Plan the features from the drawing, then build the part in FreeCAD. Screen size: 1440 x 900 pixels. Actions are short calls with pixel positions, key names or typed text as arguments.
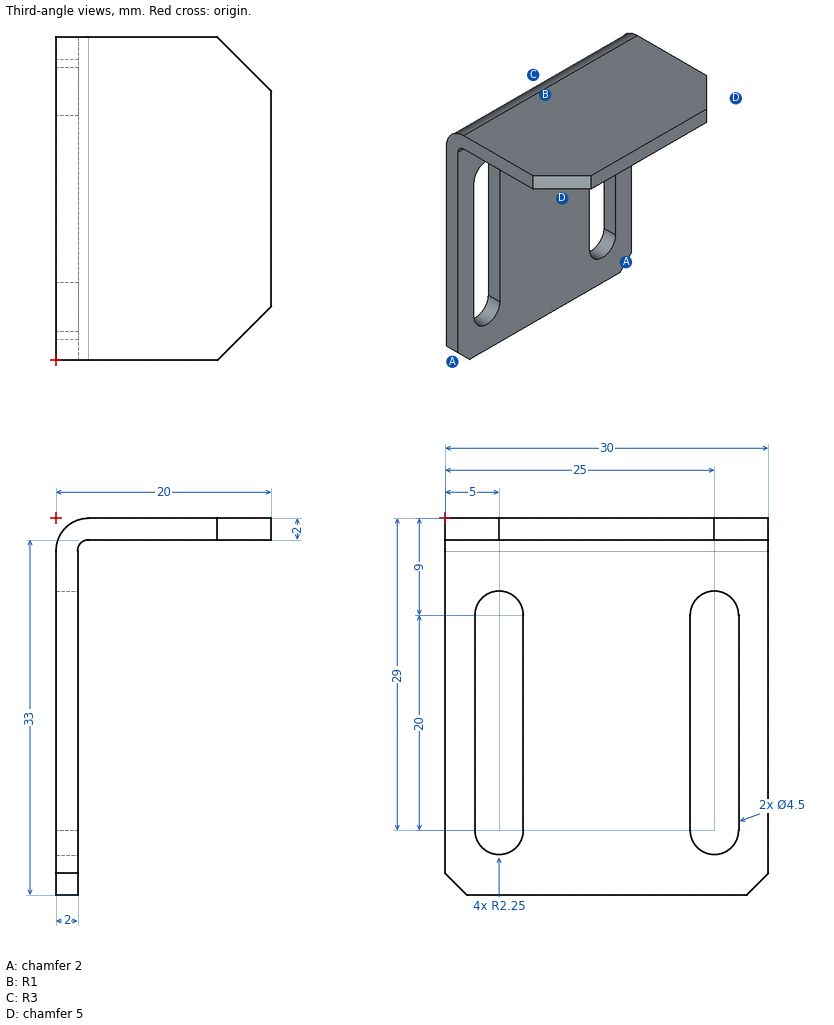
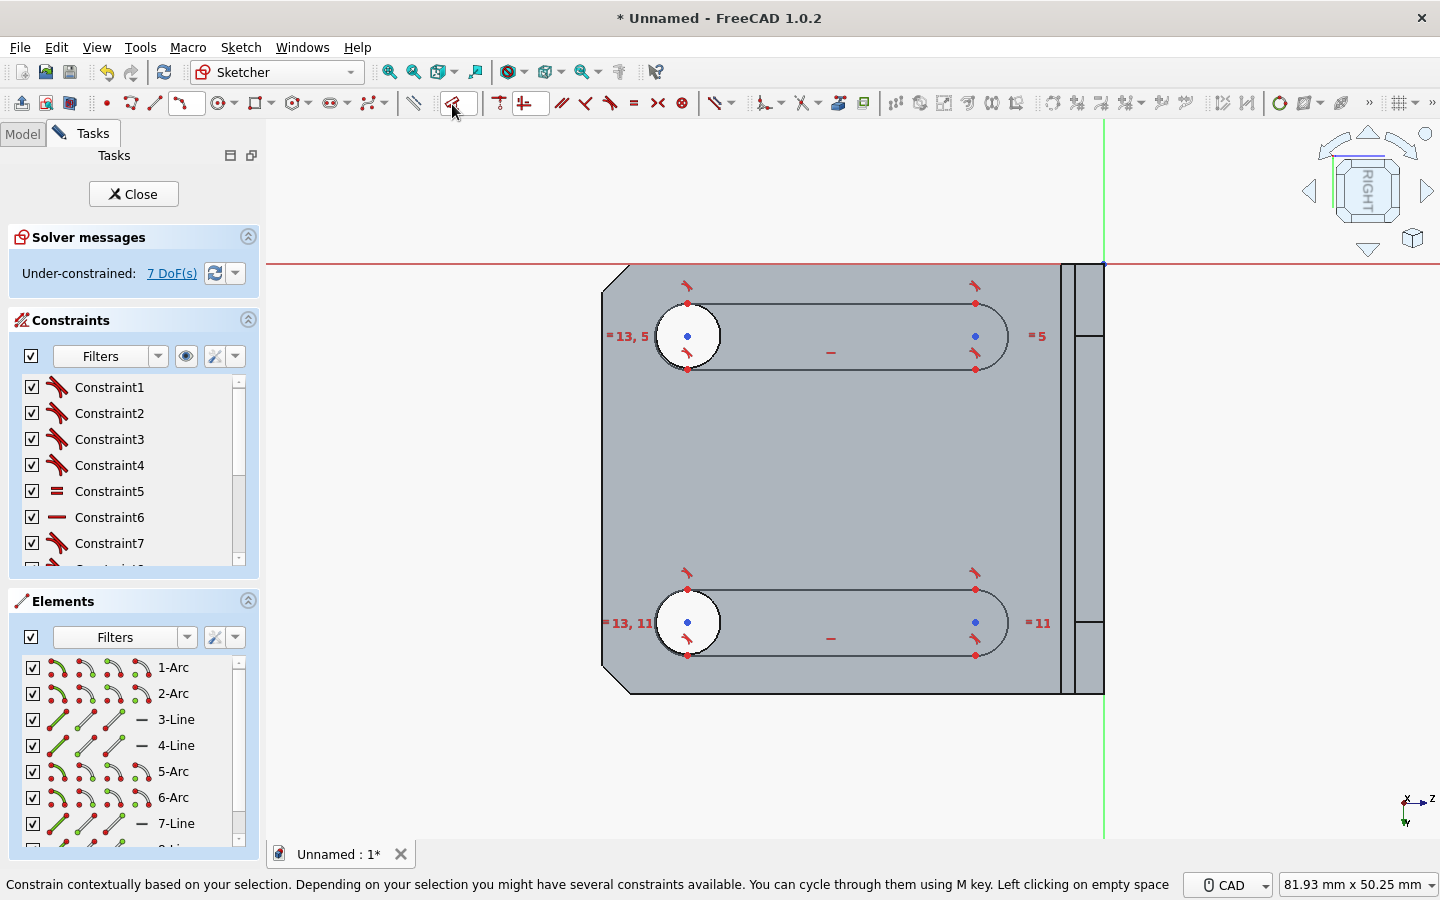
scroll(661, 318, up, 2)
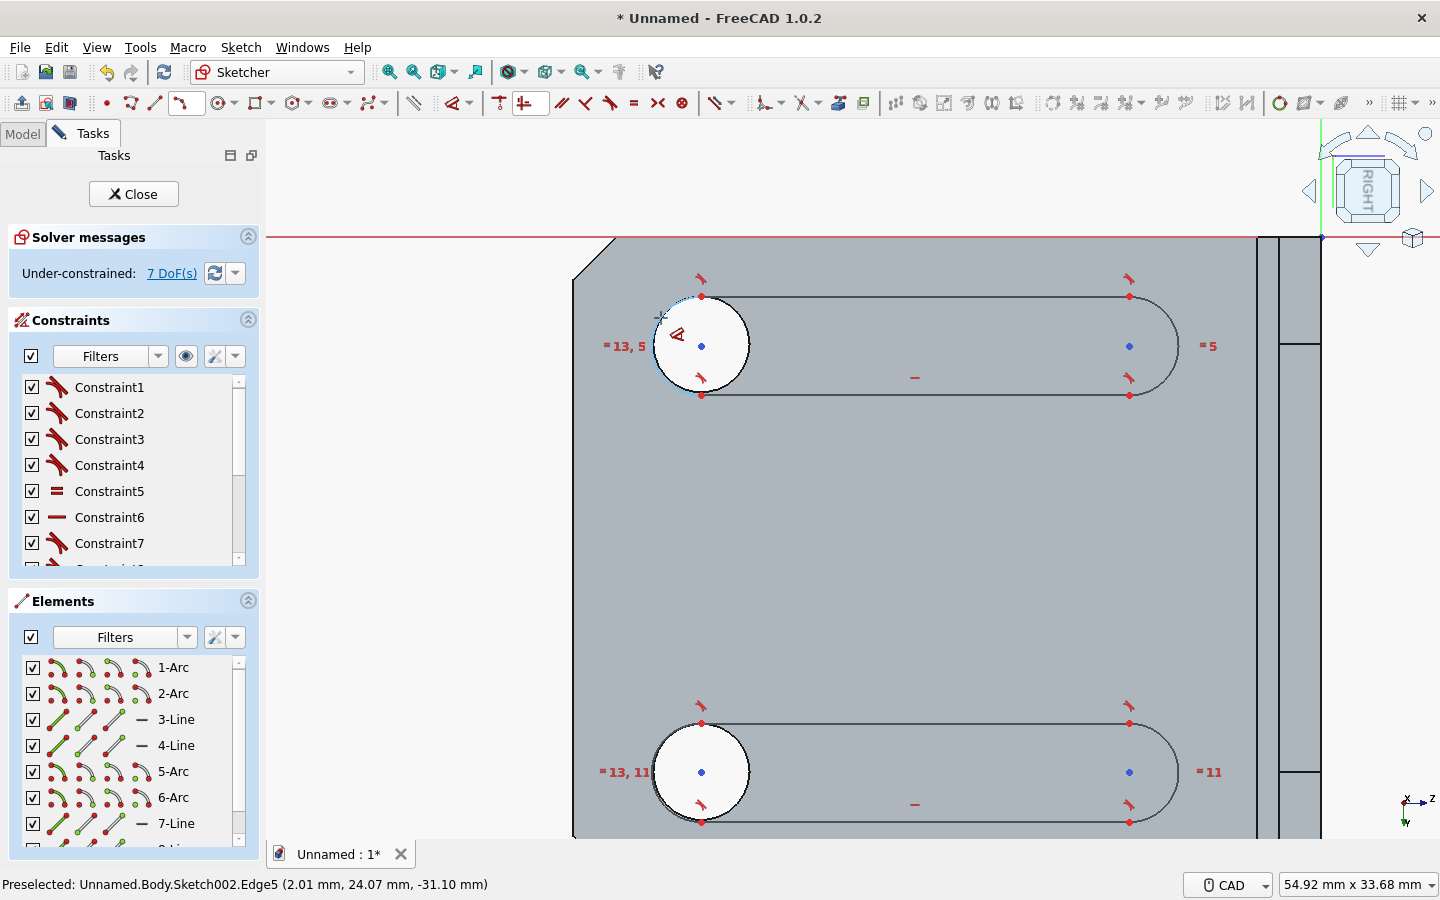
click(661, 317)
click(635, 298)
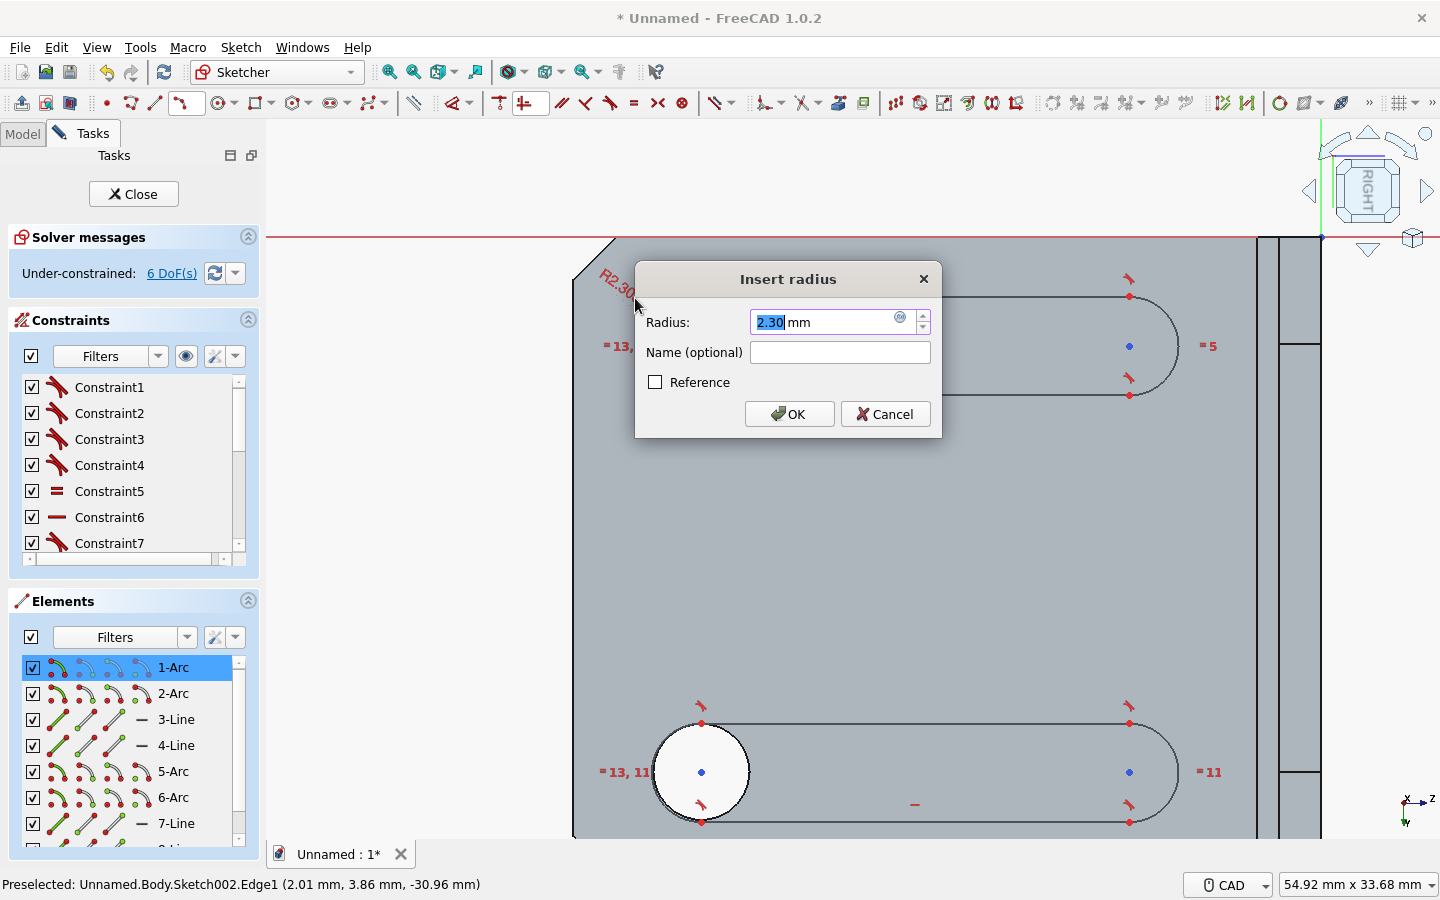
text(2.25)
key(Return)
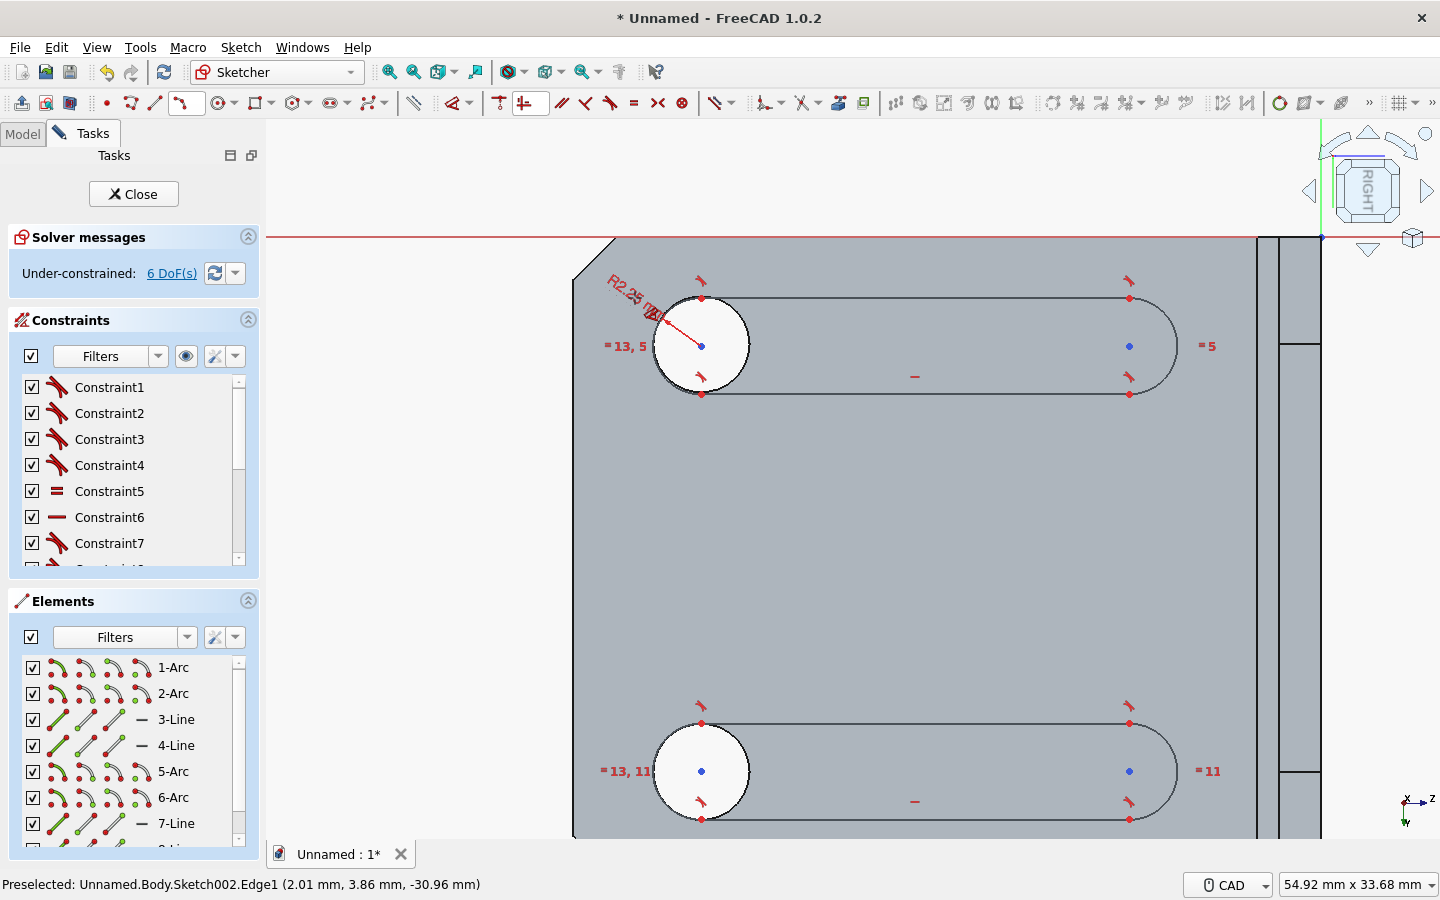
click(830, 298)
click(915, 264)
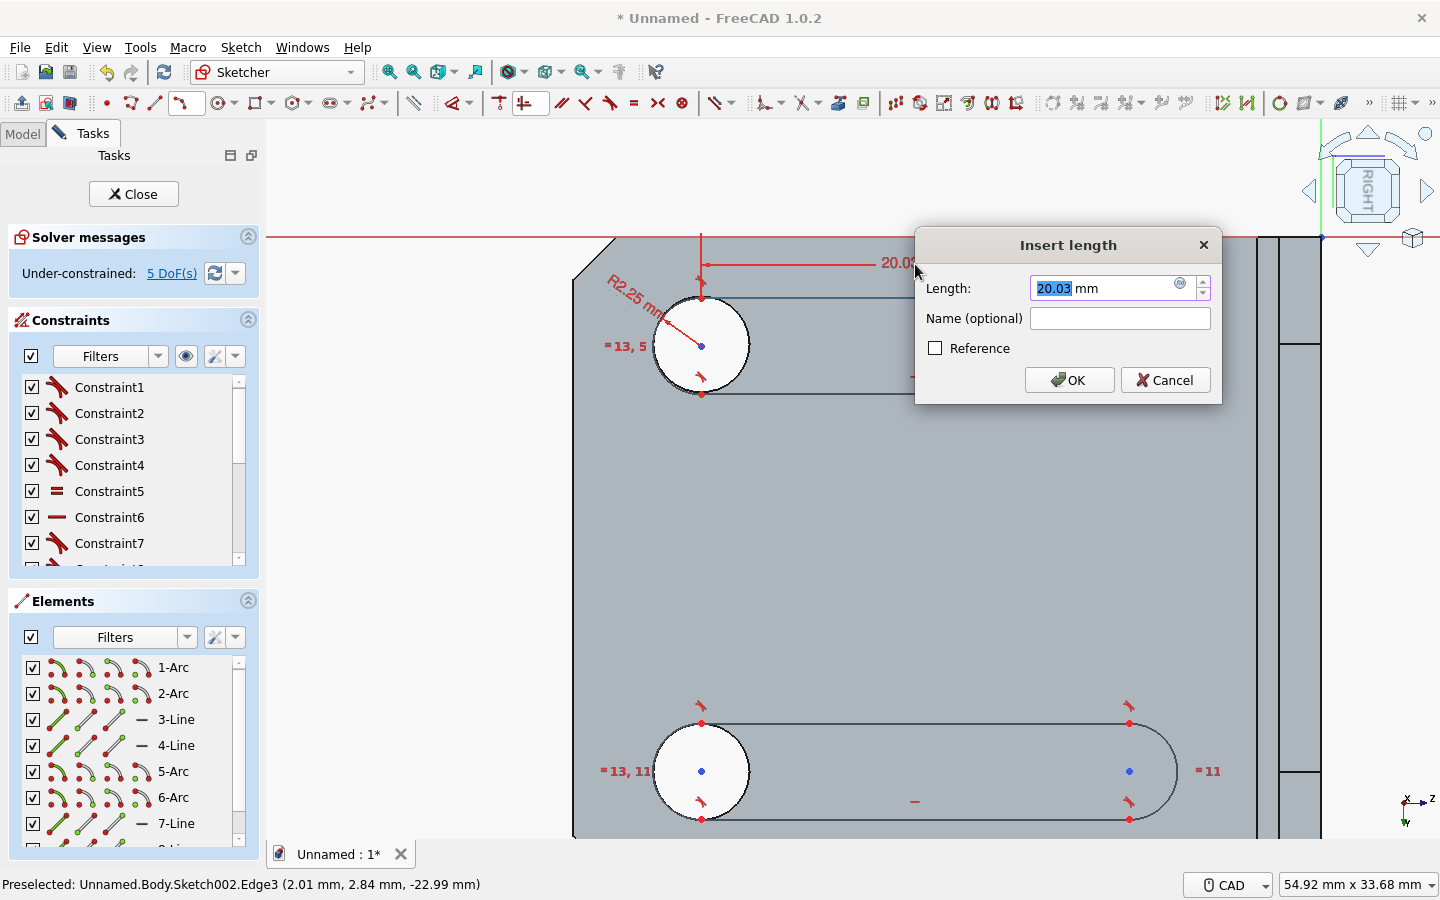
text(20)
key(Return)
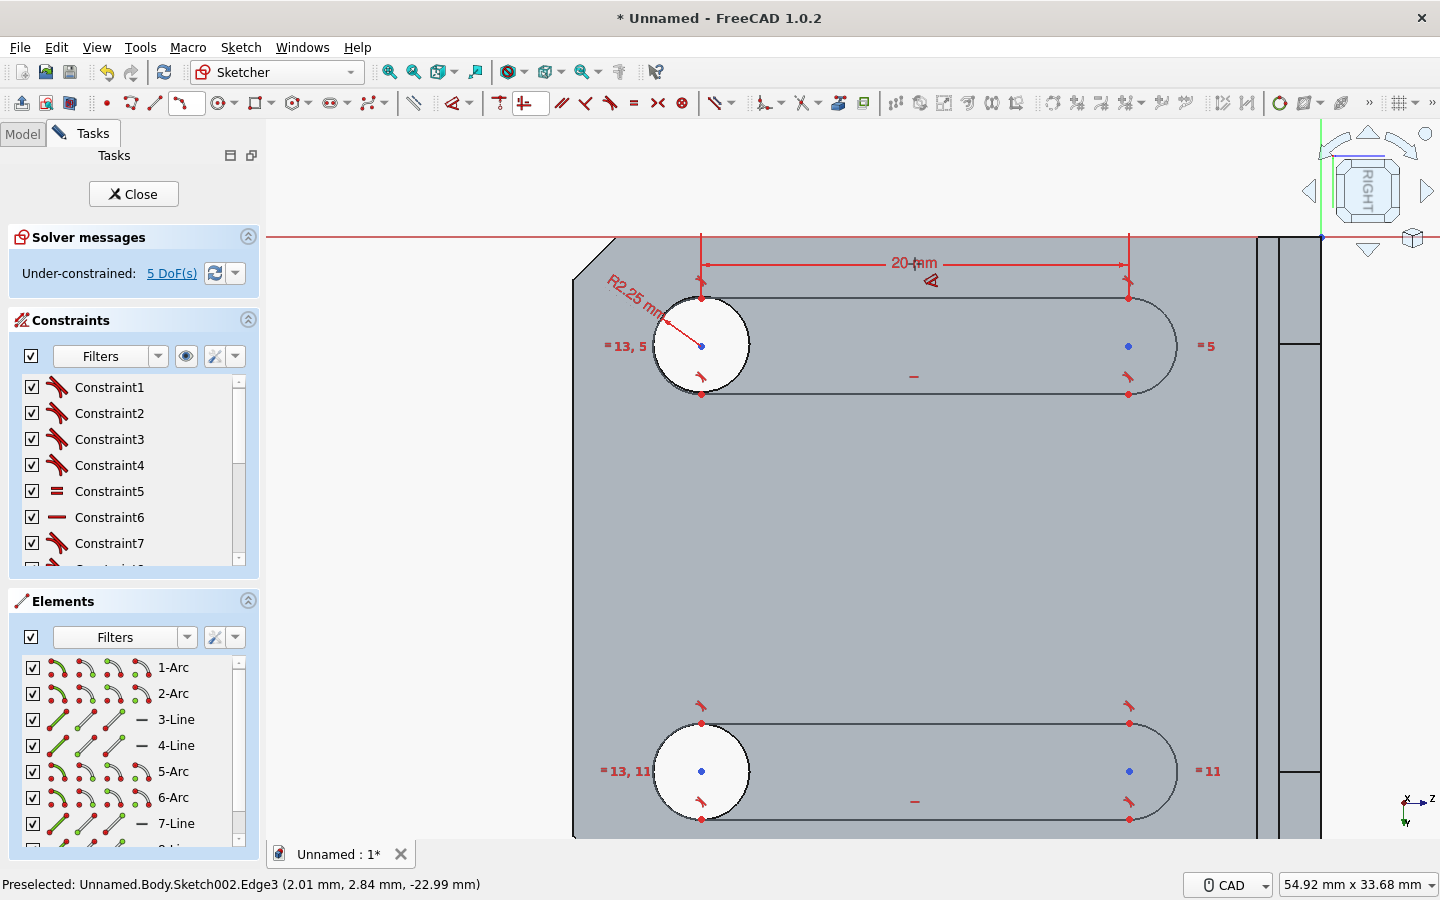
click(830, 724)
click(915, 758)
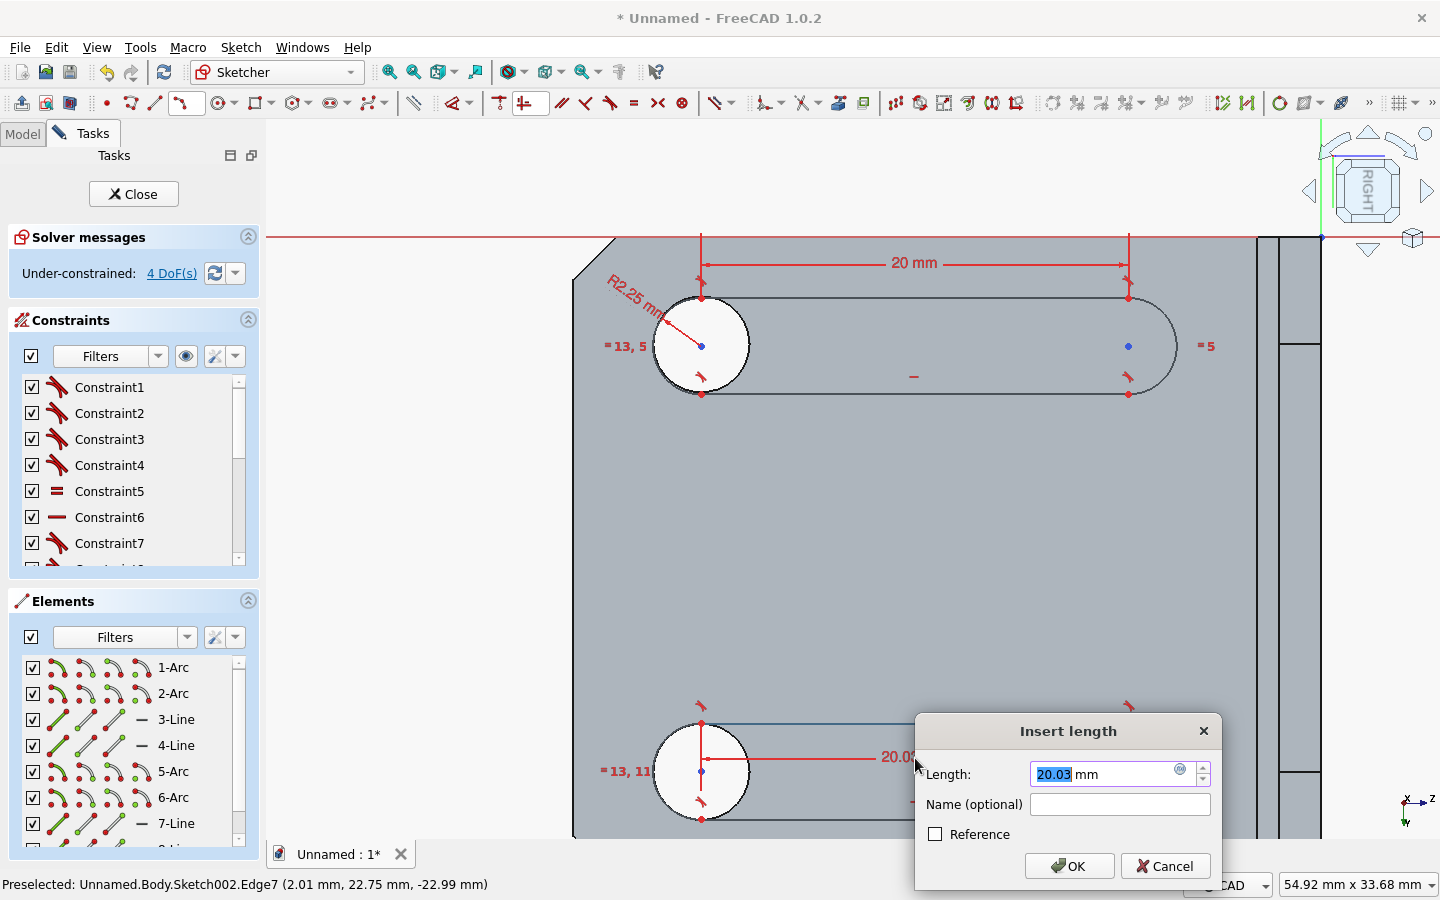
text(20)
key(Return)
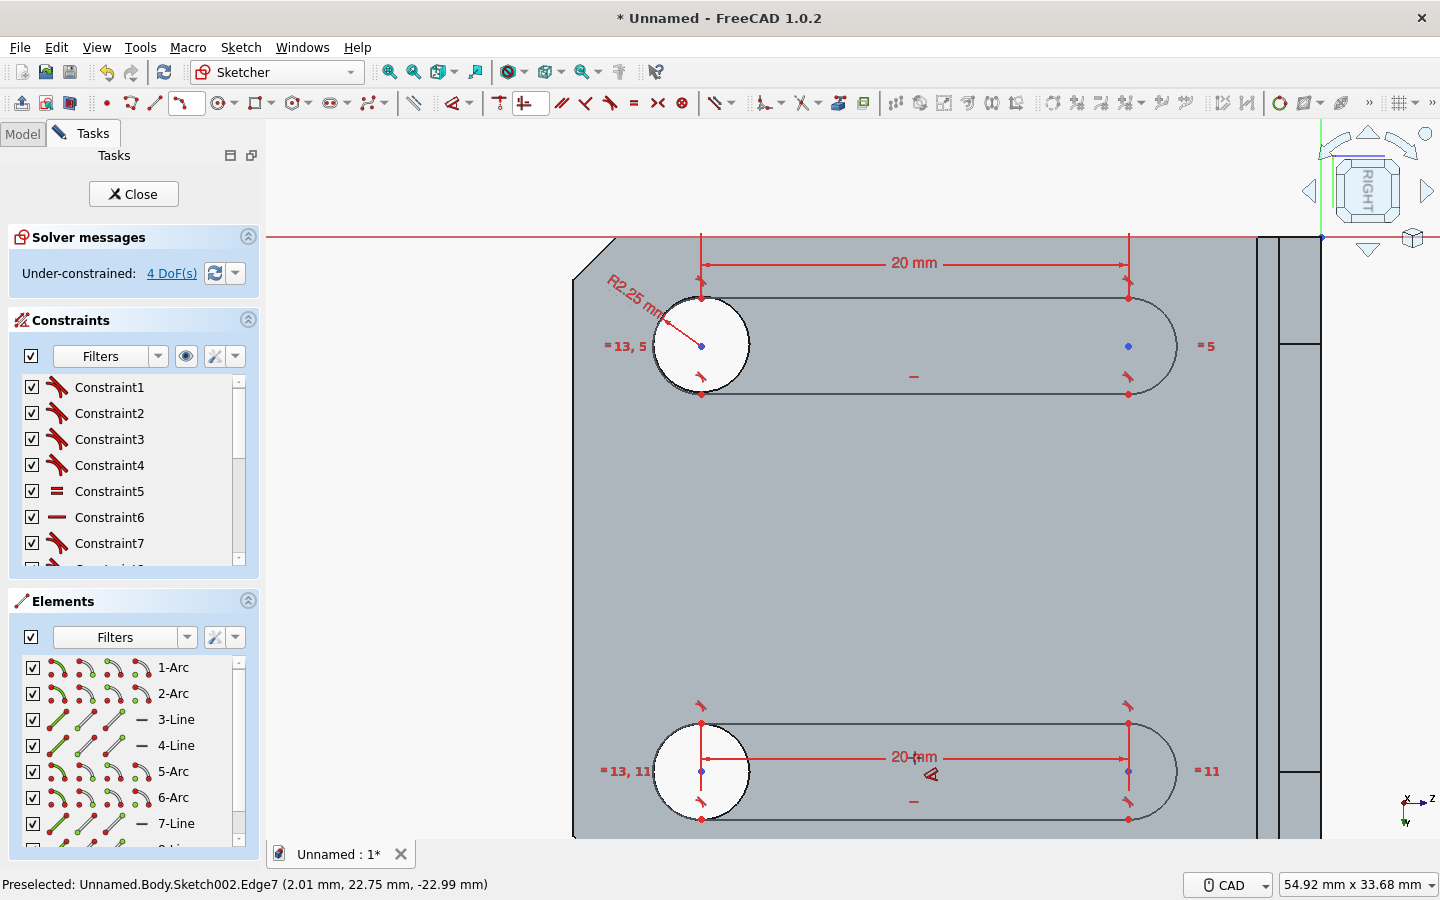
click(1129, 394)
click(1202, 203)